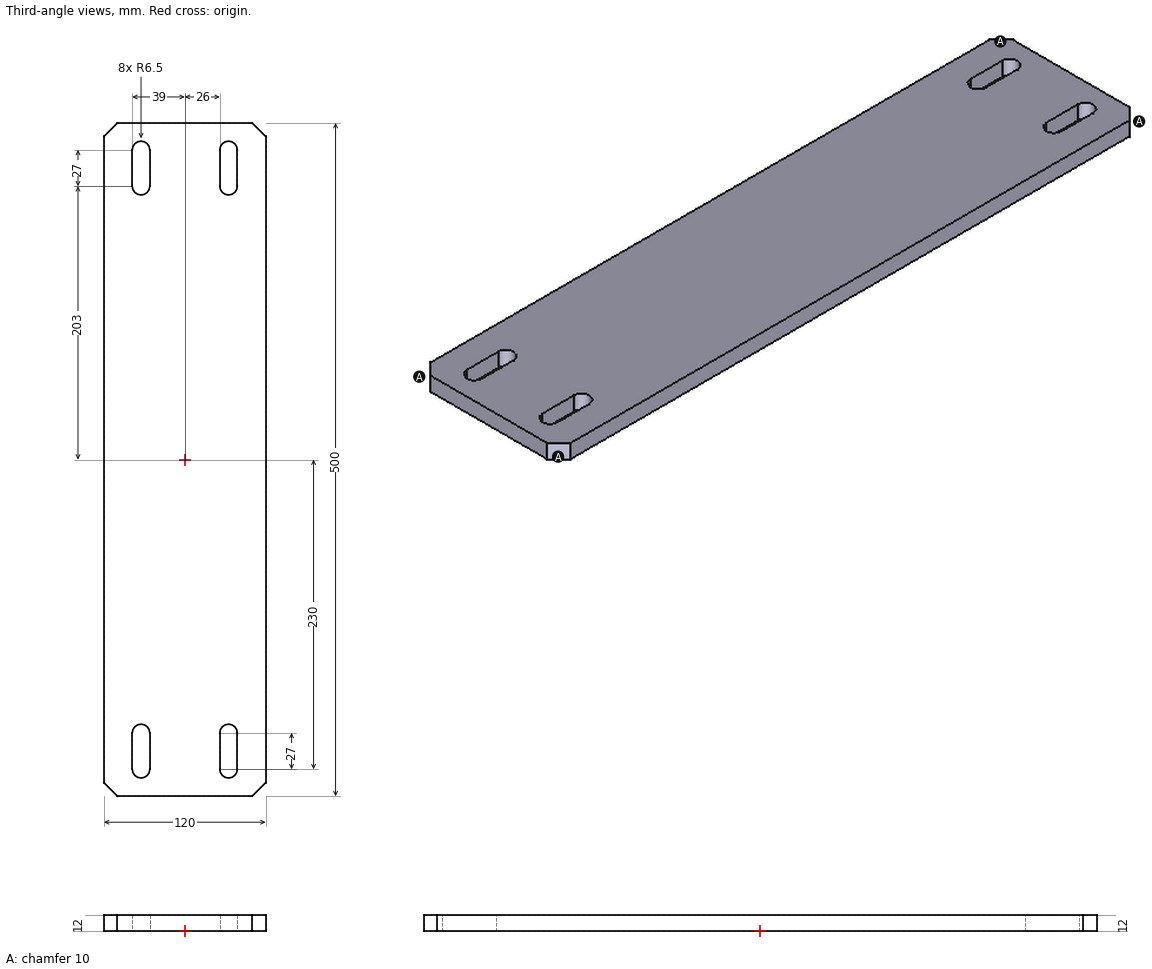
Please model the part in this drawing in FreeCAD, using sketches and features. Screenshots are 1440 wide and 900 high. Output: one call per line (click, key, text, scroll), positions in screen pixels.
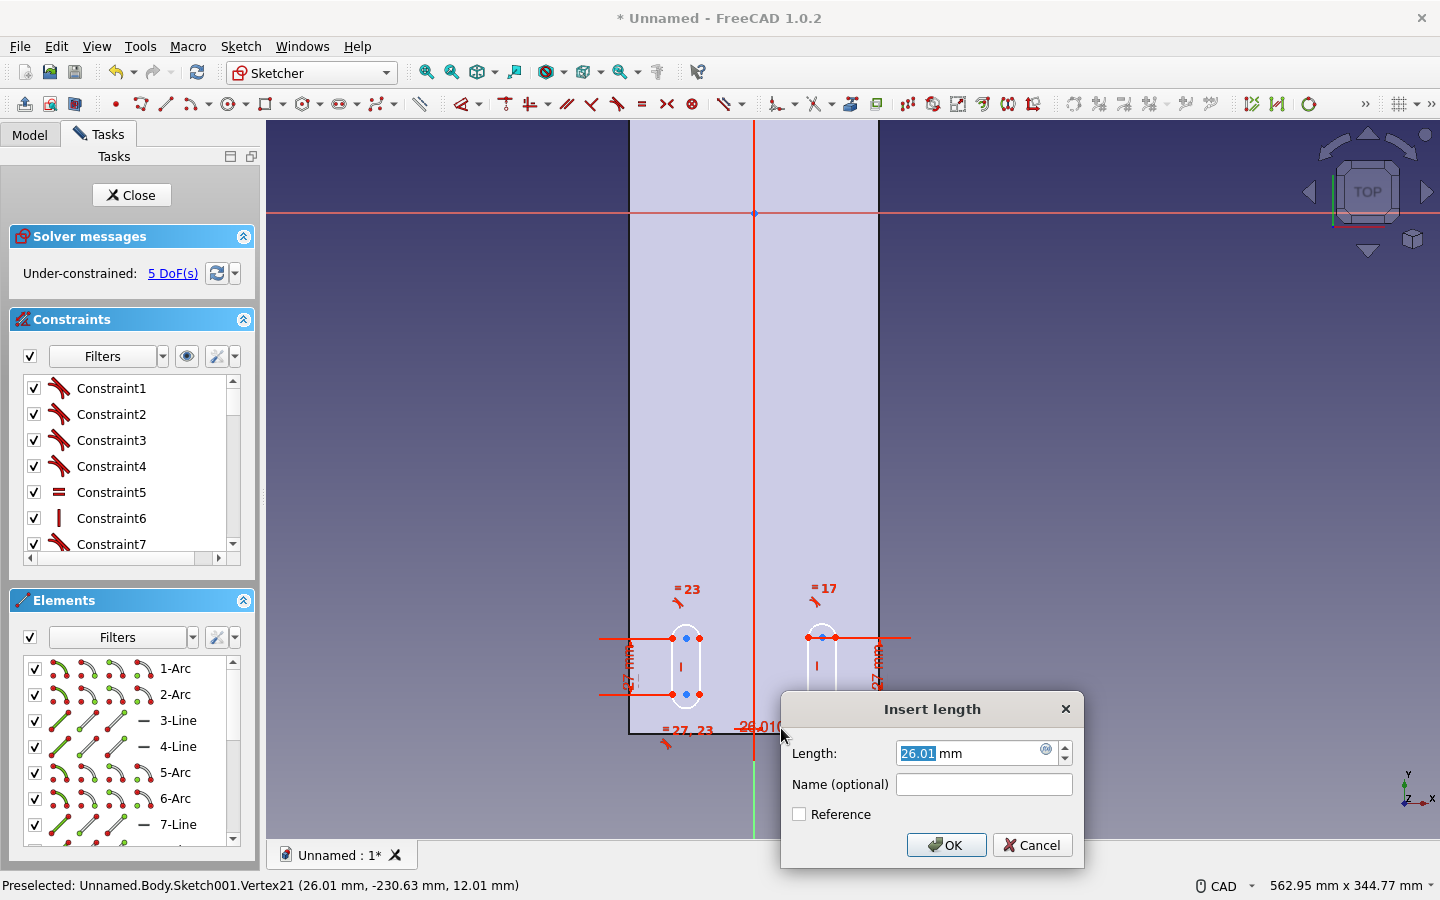
text(26)
key(Return)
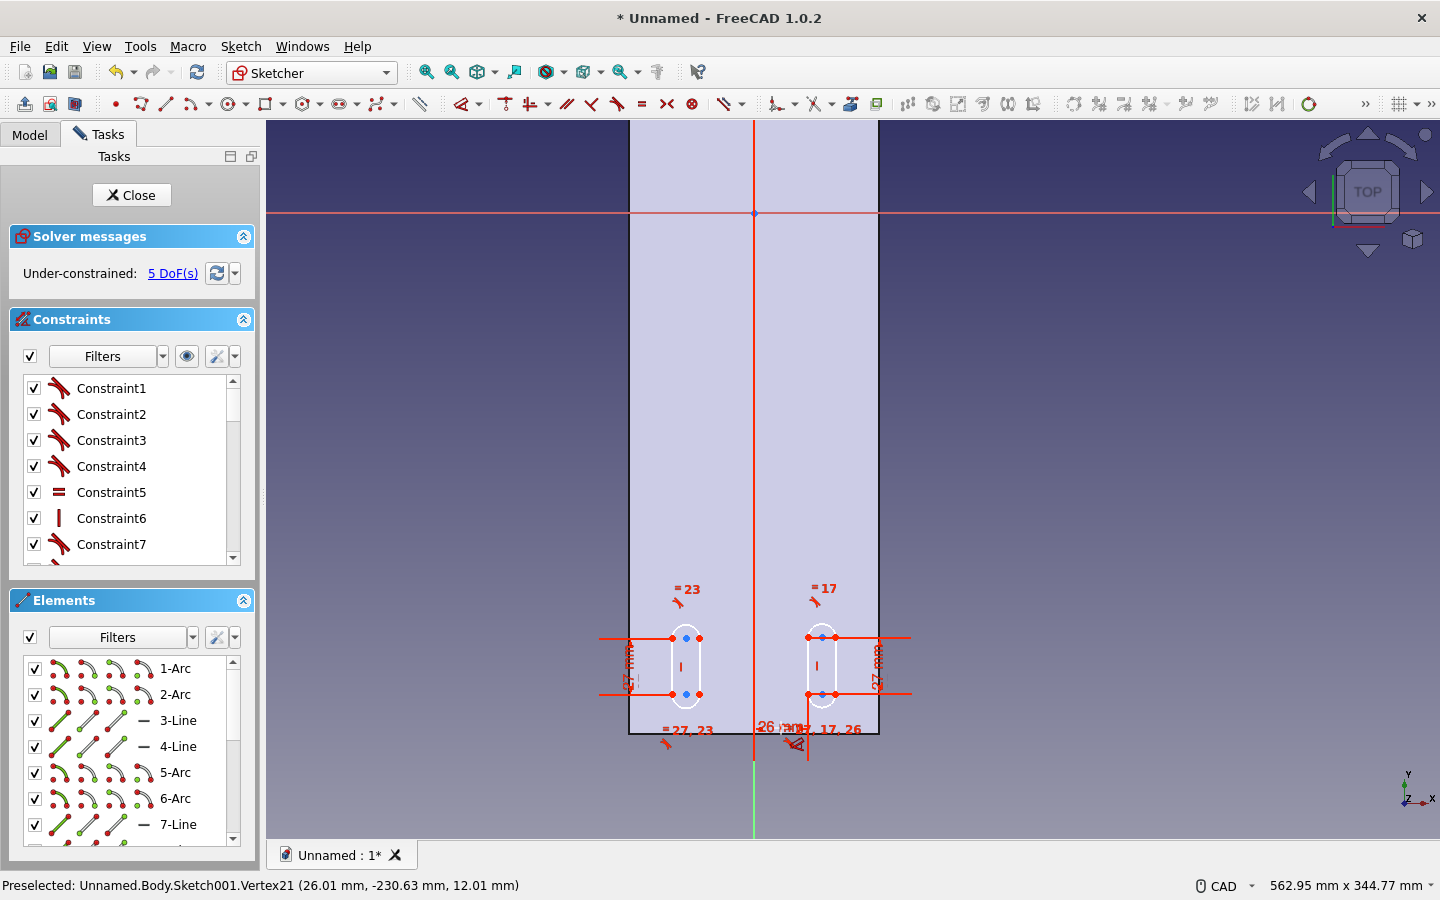
click(672, 695)
click(695, 729)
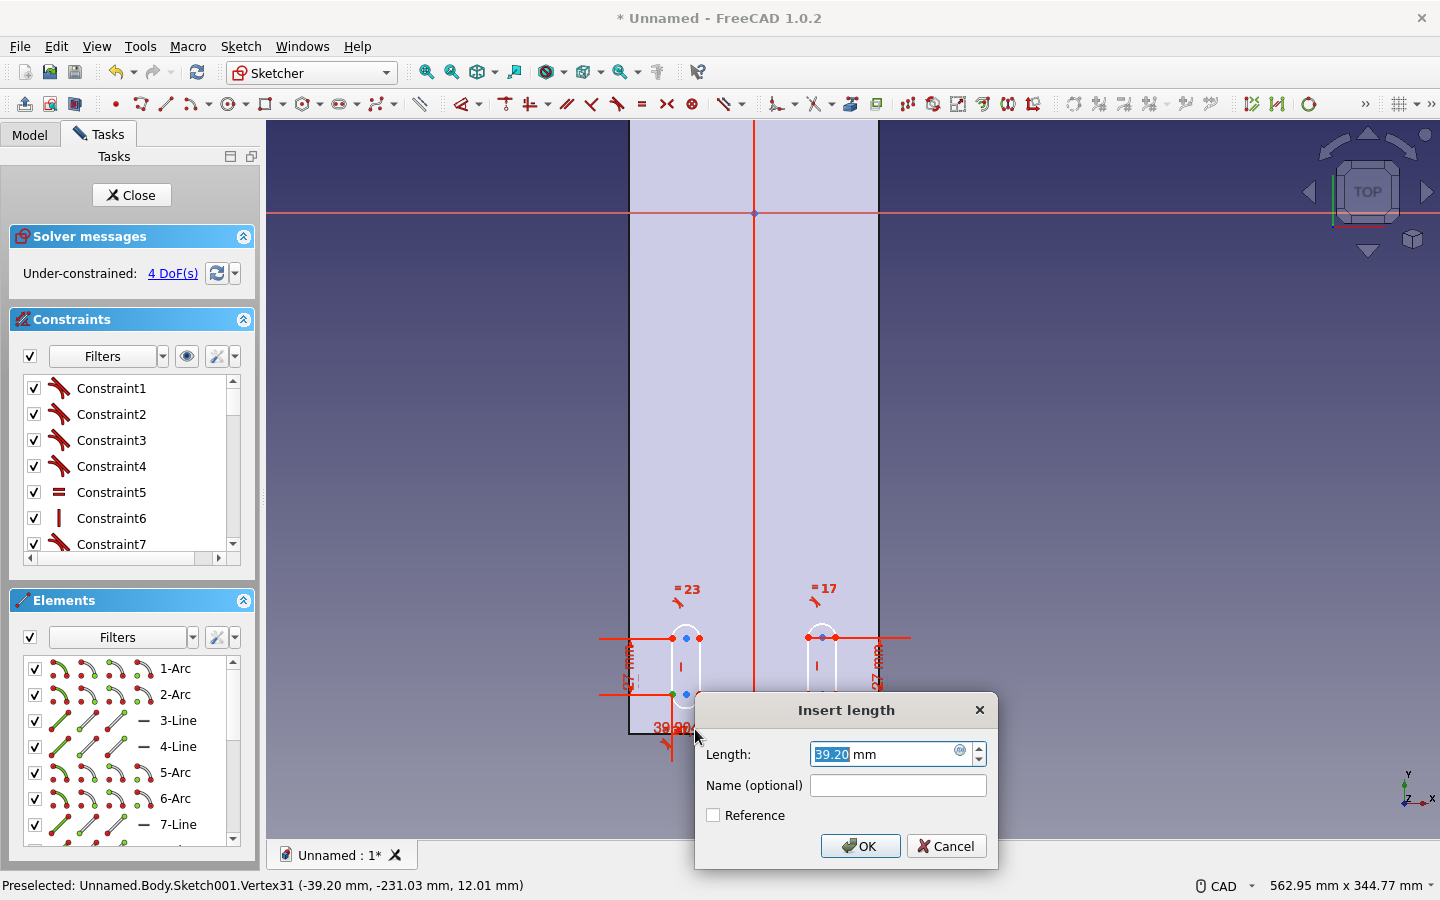
text(39)
key(Return)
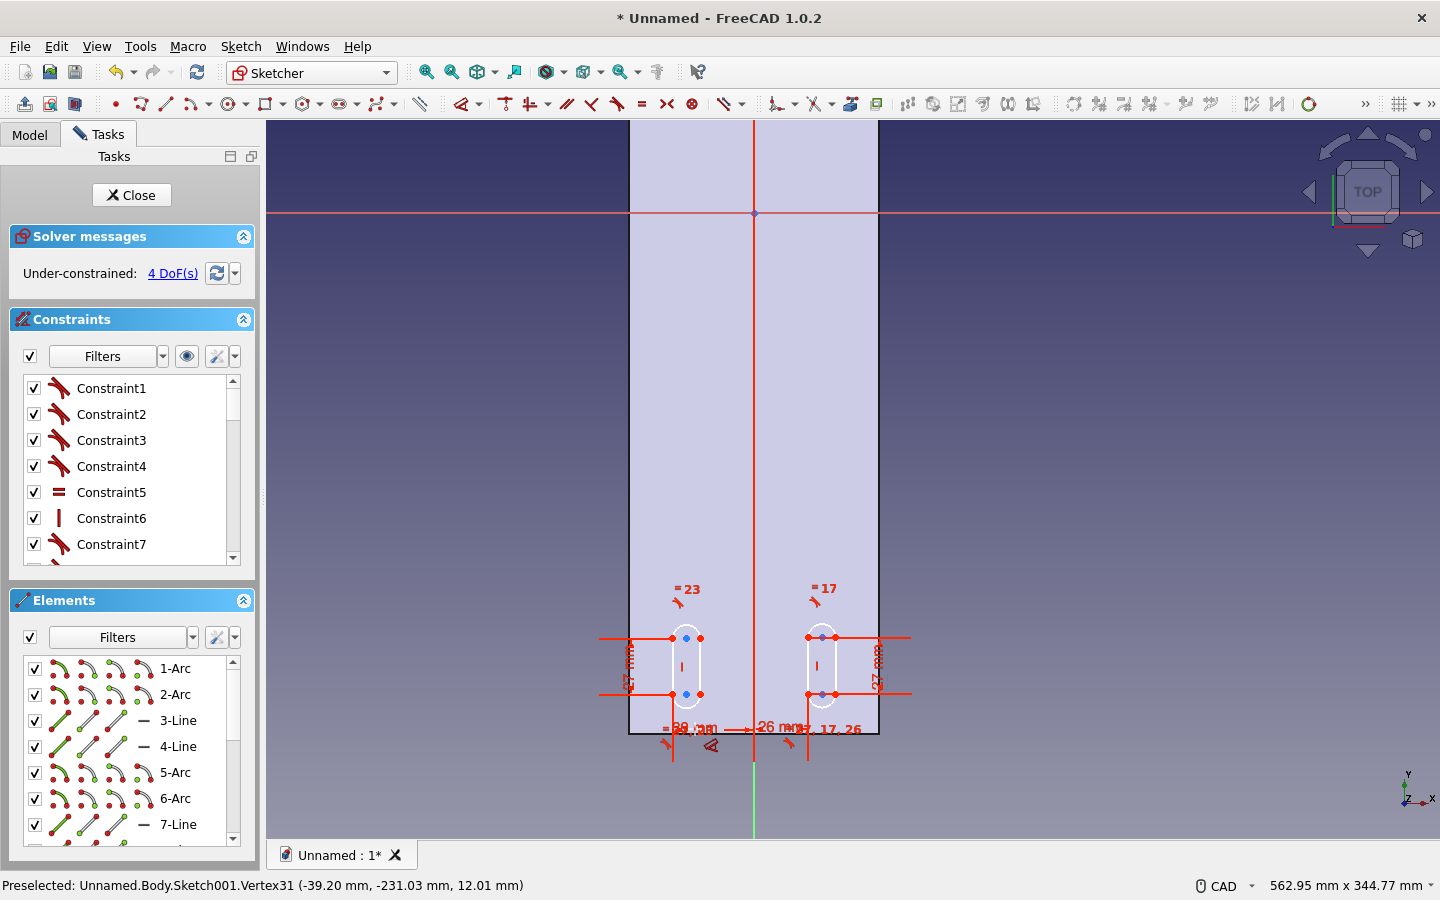
scroll(809, 697, down, 4)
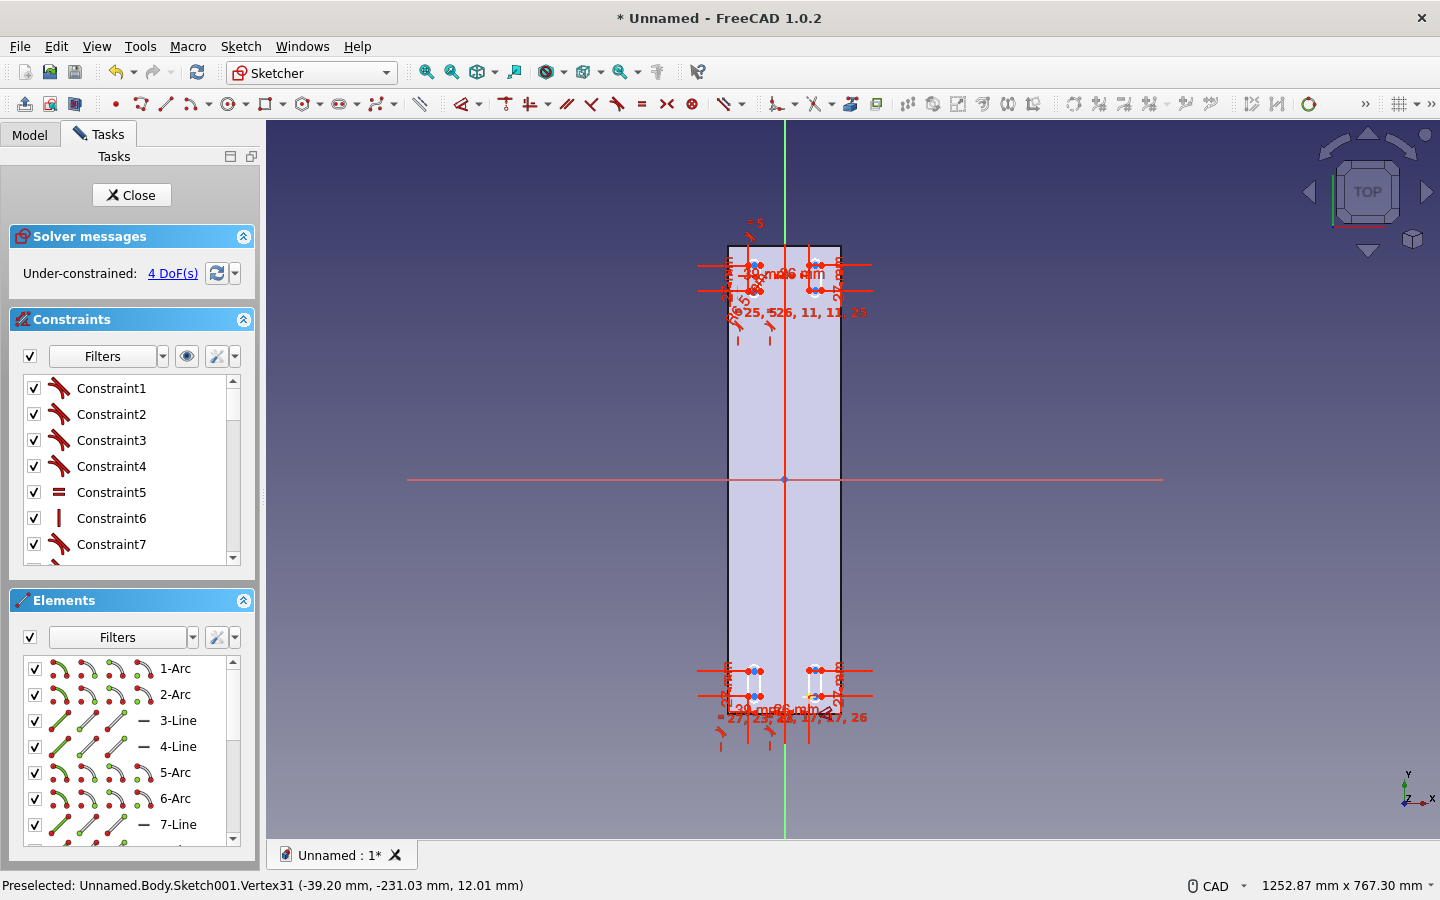
scroll(748, 291, up, 4)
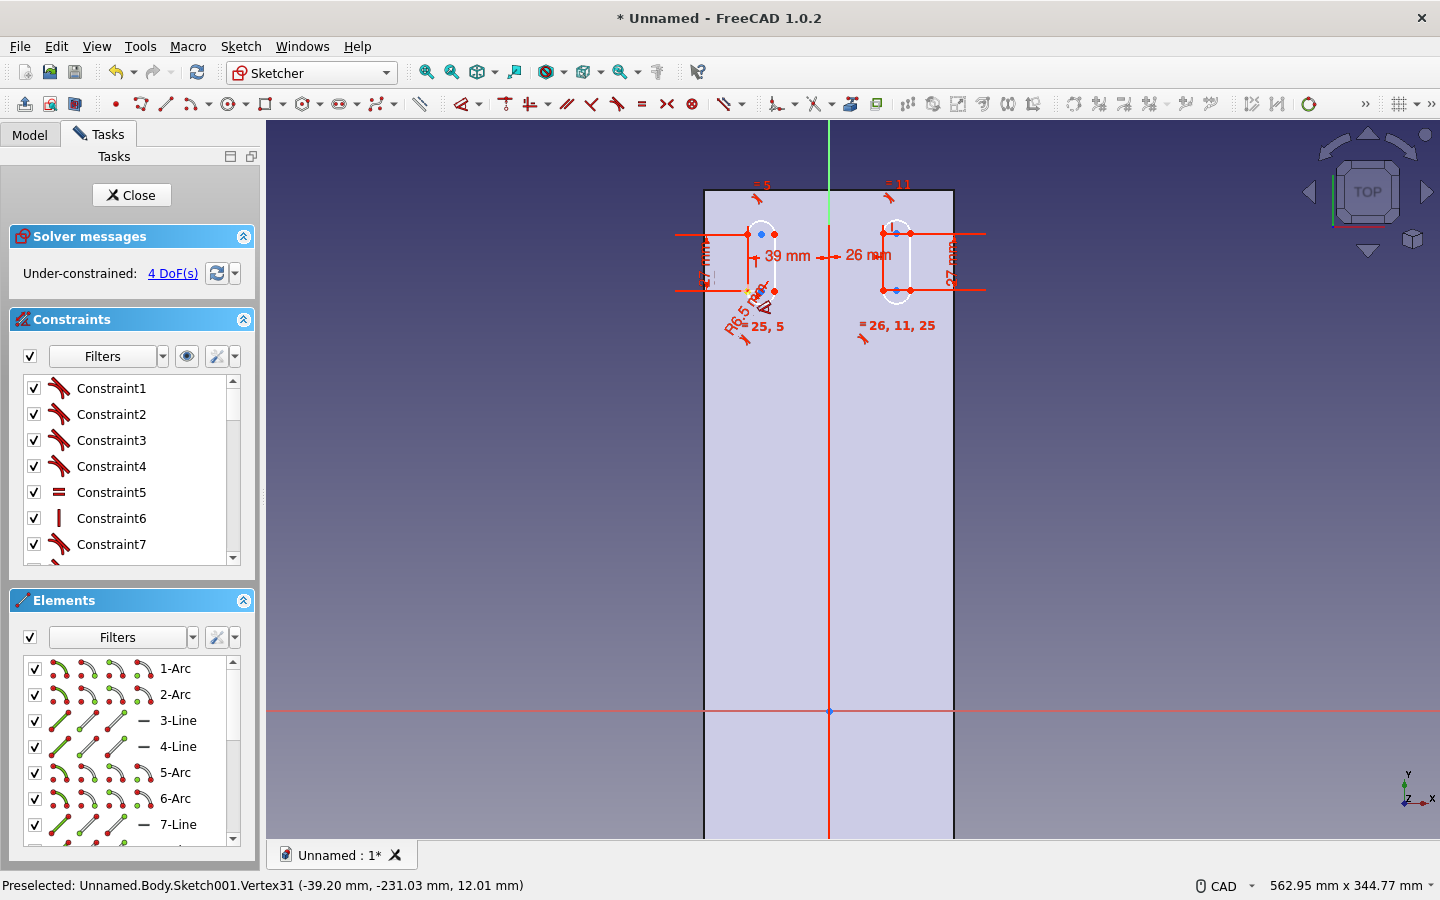
click(748, 291)
click(714, 501)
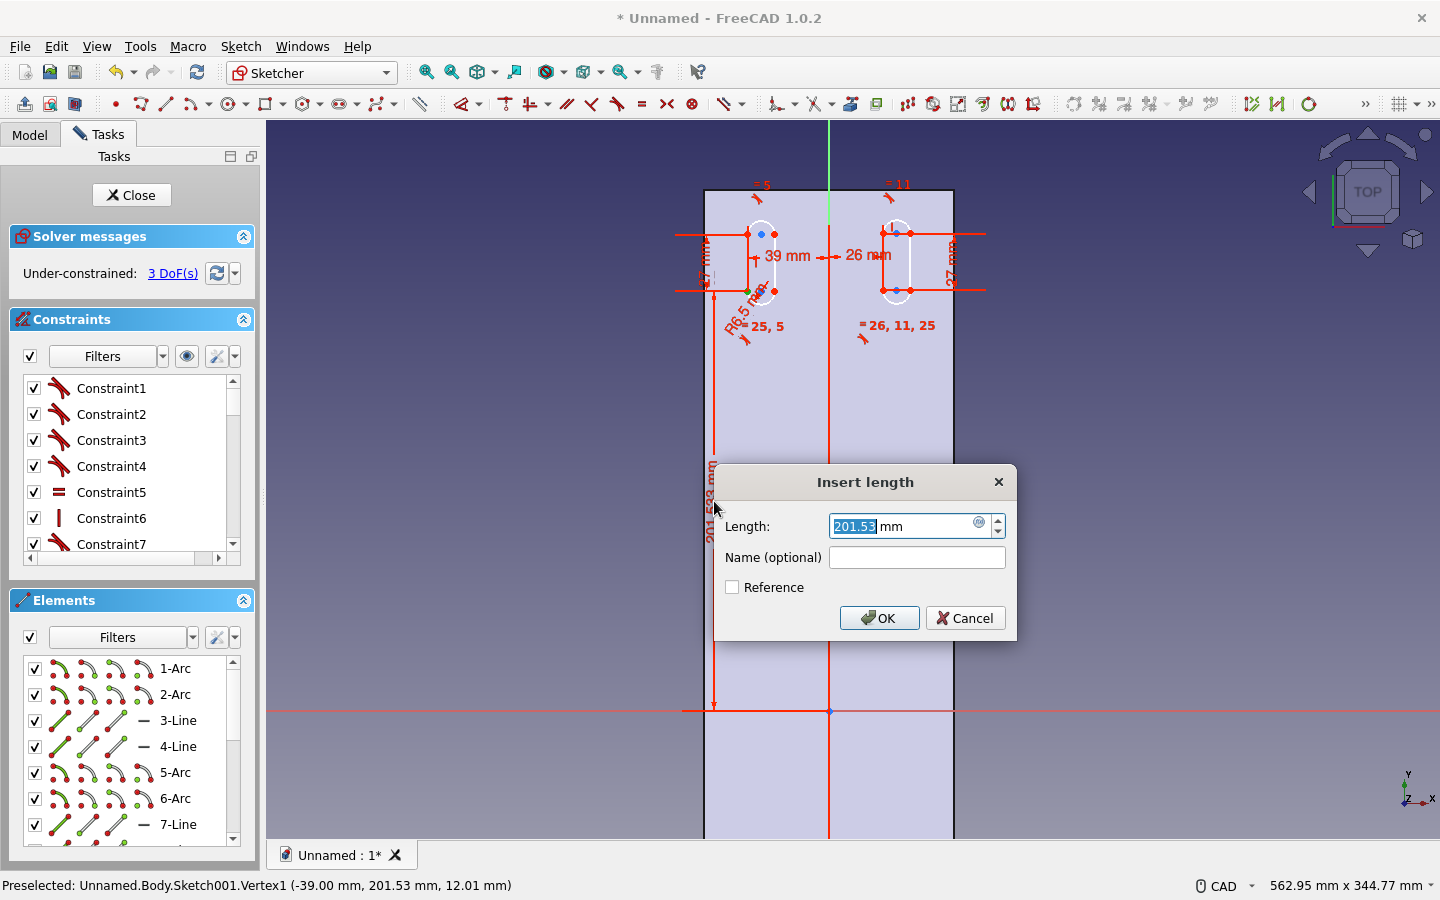
text(203)
key(Return)